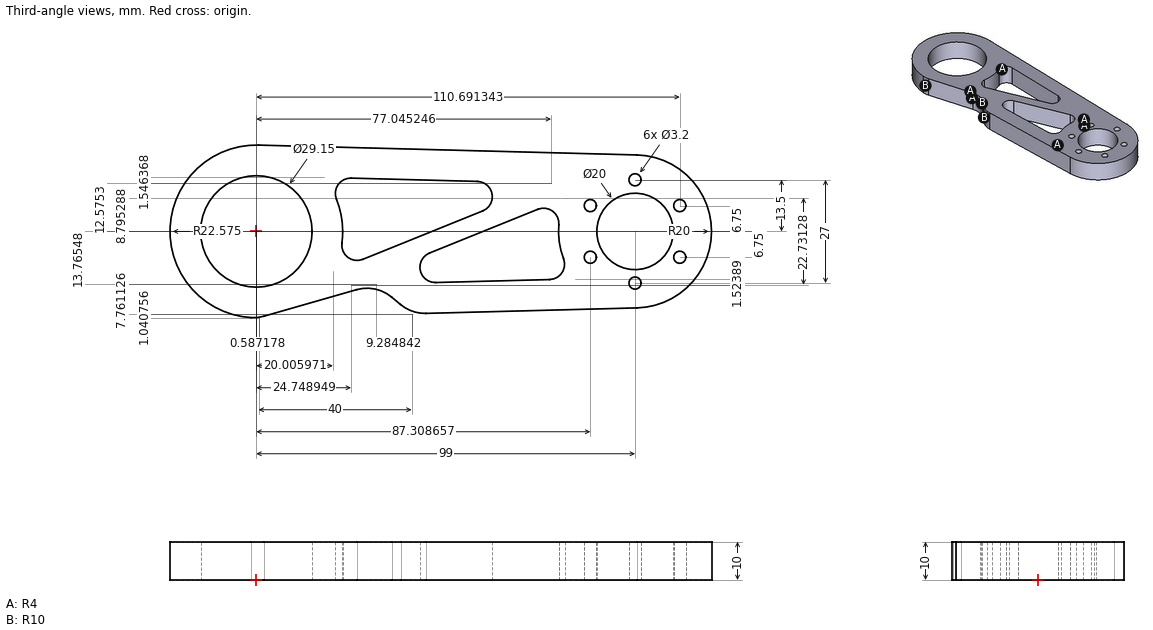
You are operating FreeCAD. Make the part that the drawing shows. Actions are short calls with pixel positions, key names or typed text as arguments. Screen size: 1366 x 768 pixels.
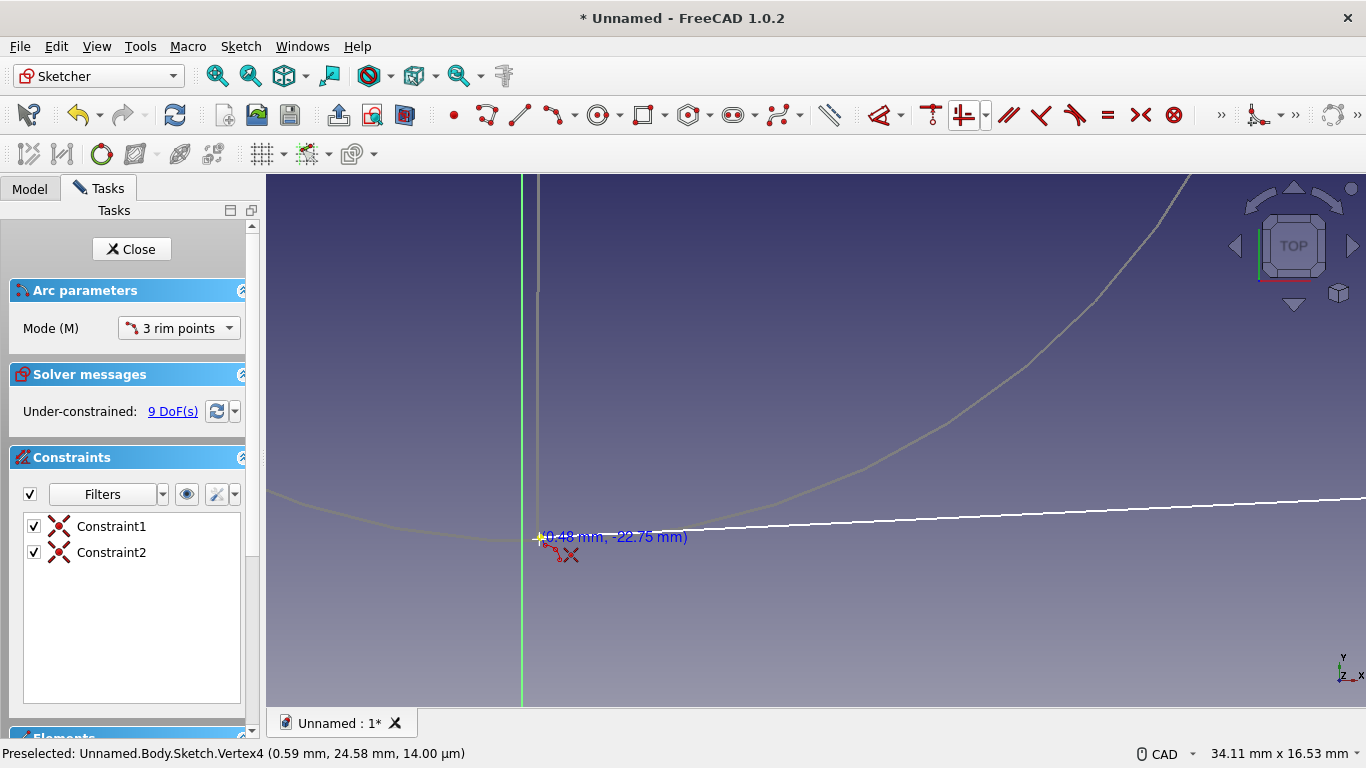
click(541, 537)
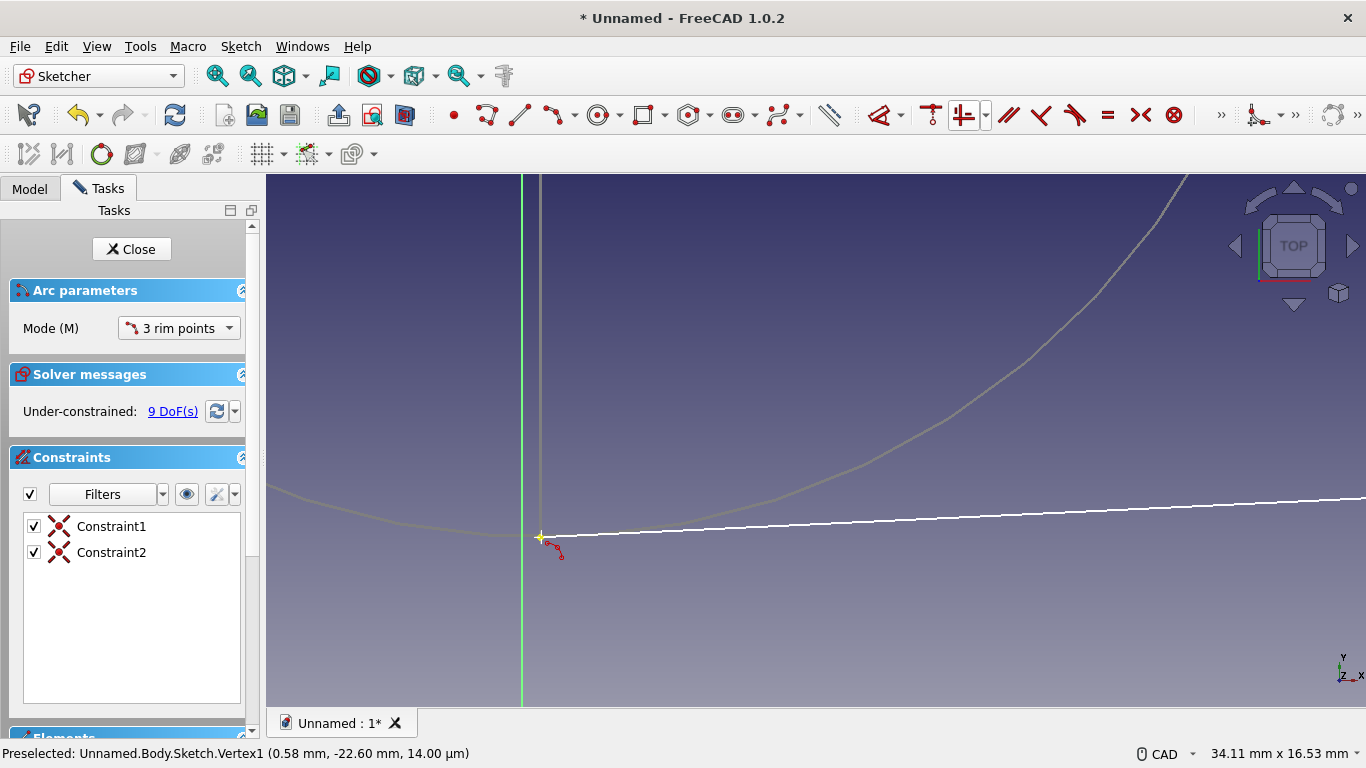
scroll(539, 539, down, 10)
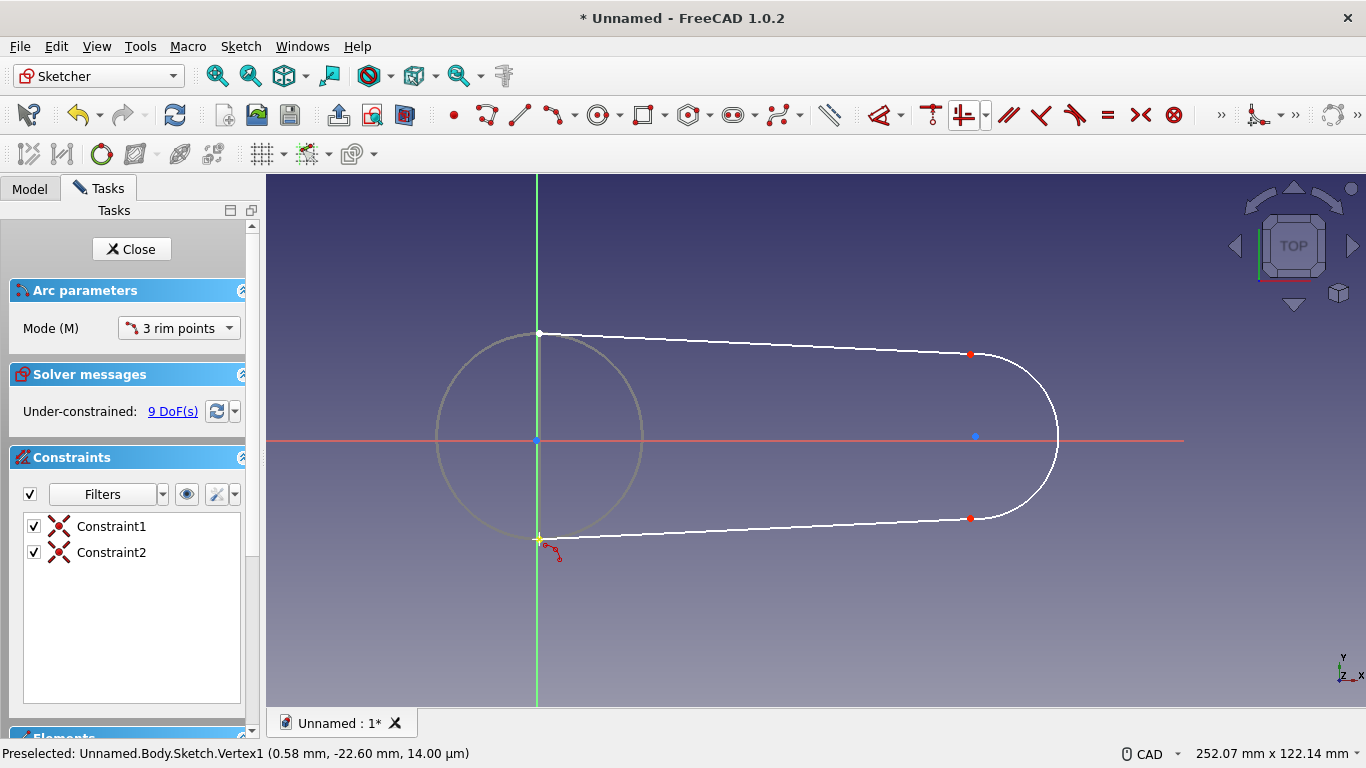
click(443, 410)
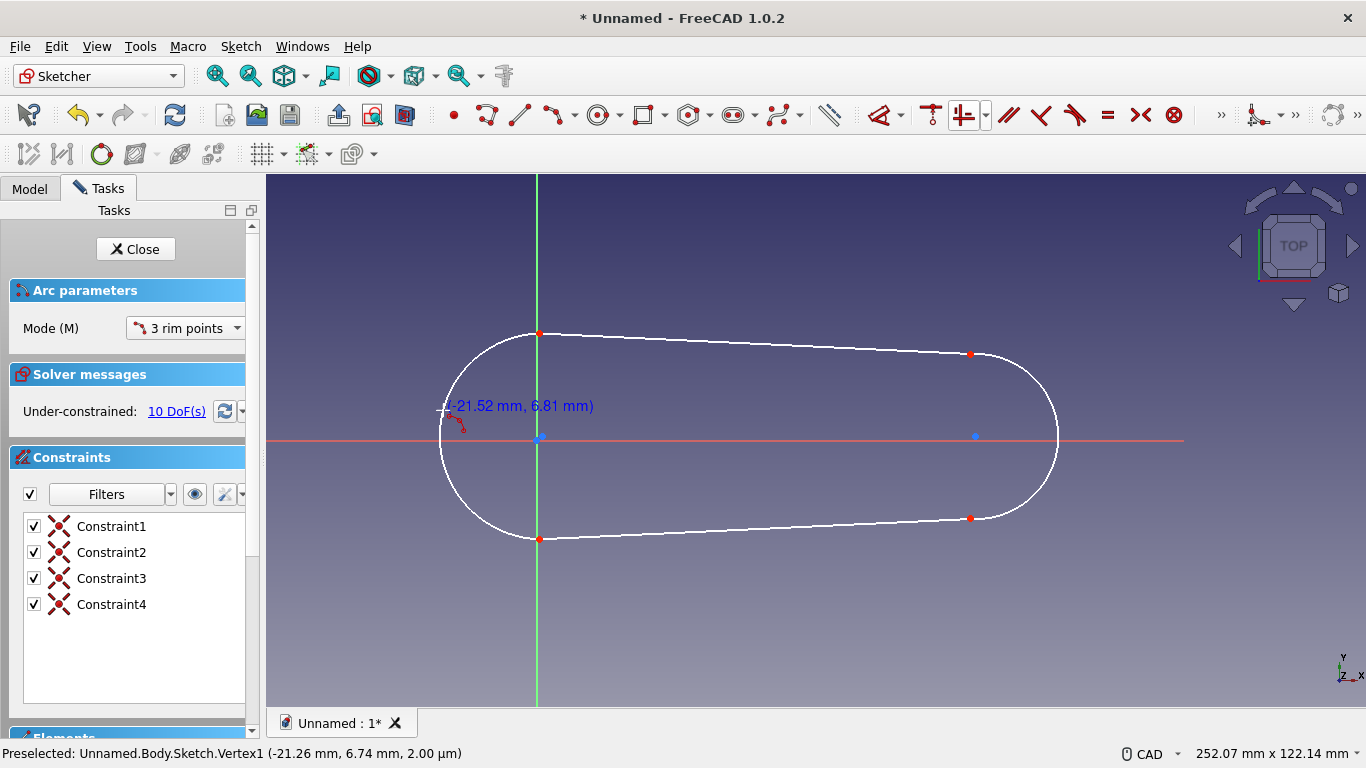
key(g)
key(c)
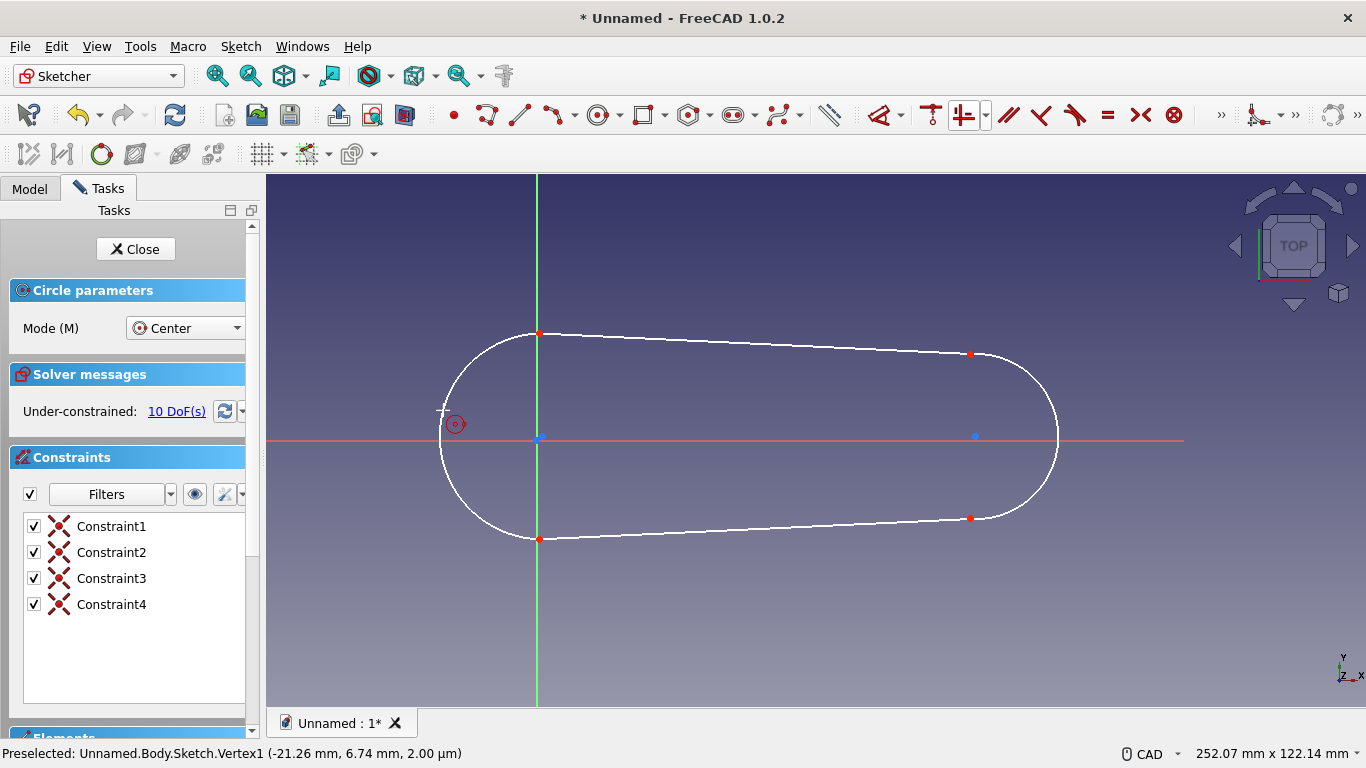
click(537, 441)
move(582, 396)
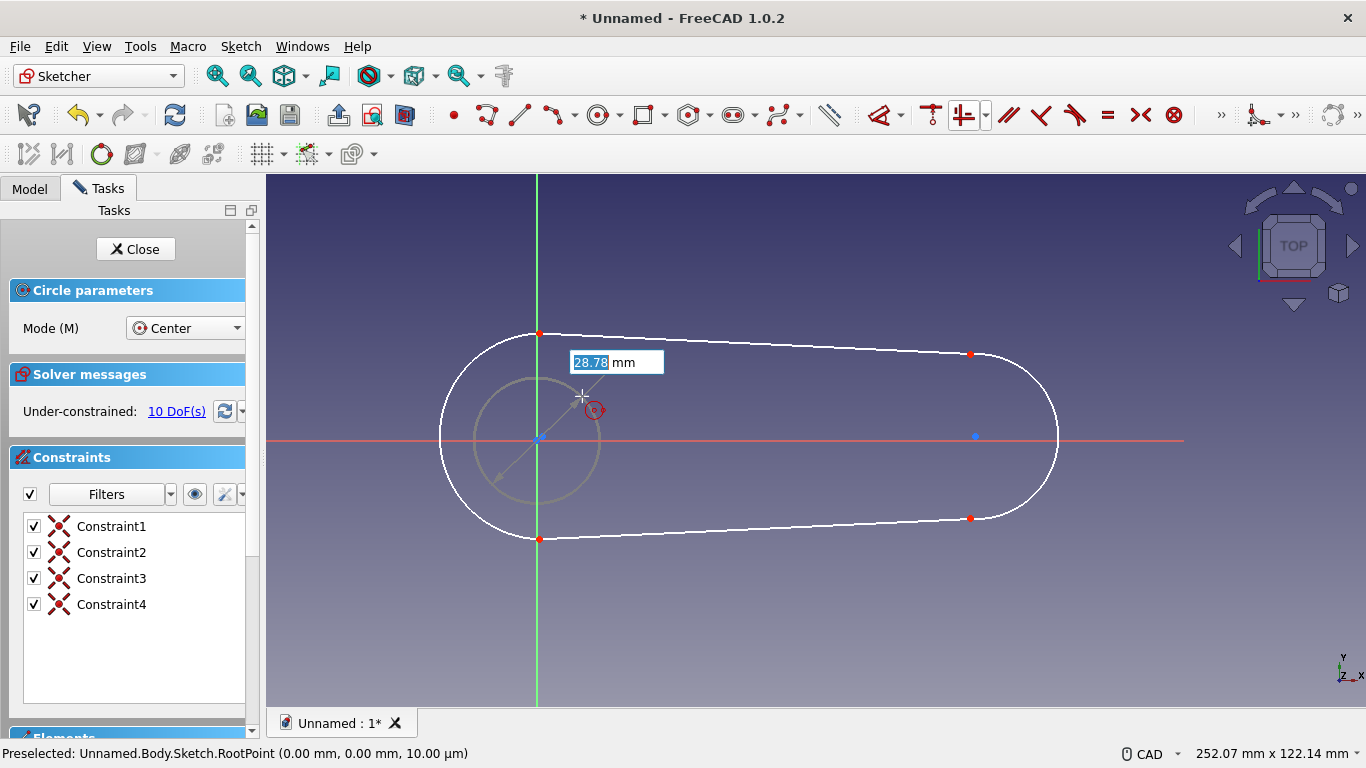
text(29.15)
key(Return)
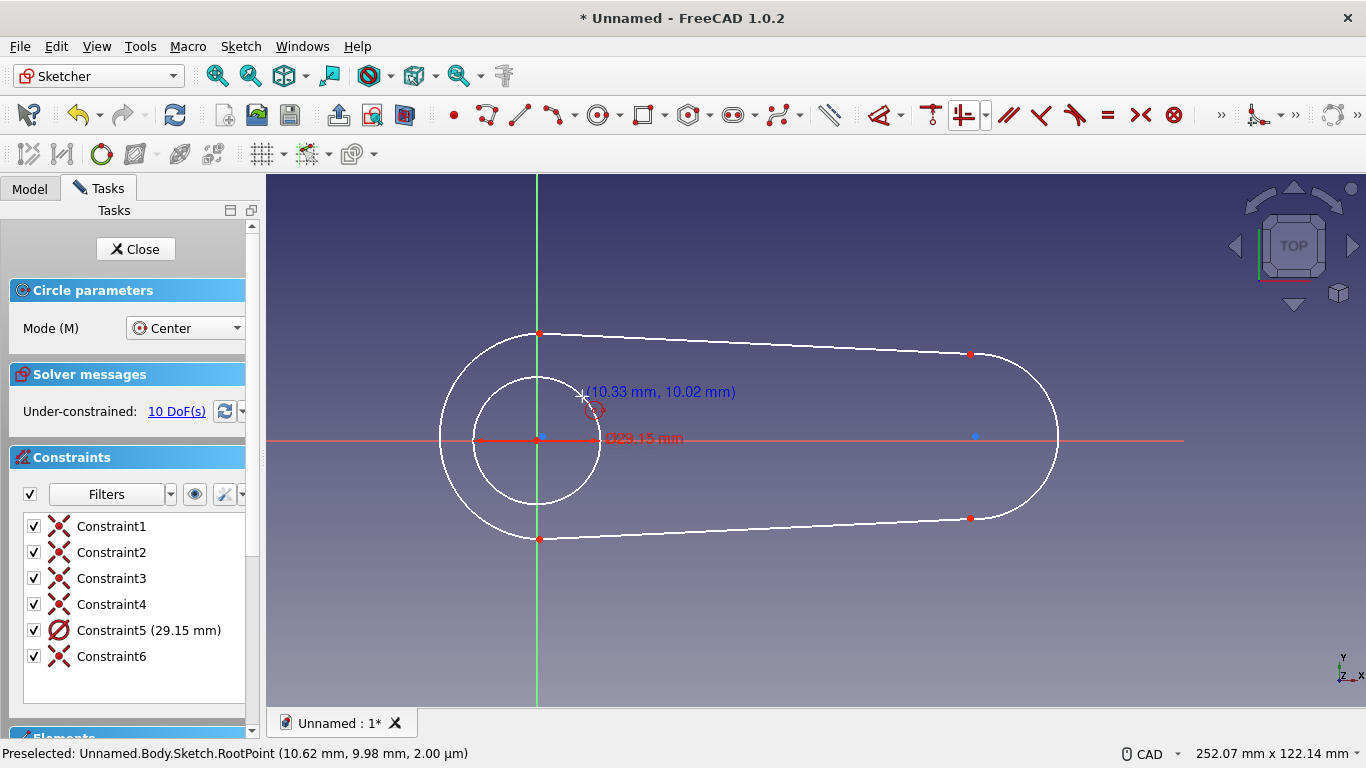
click(969, 441)
move(1000, 410)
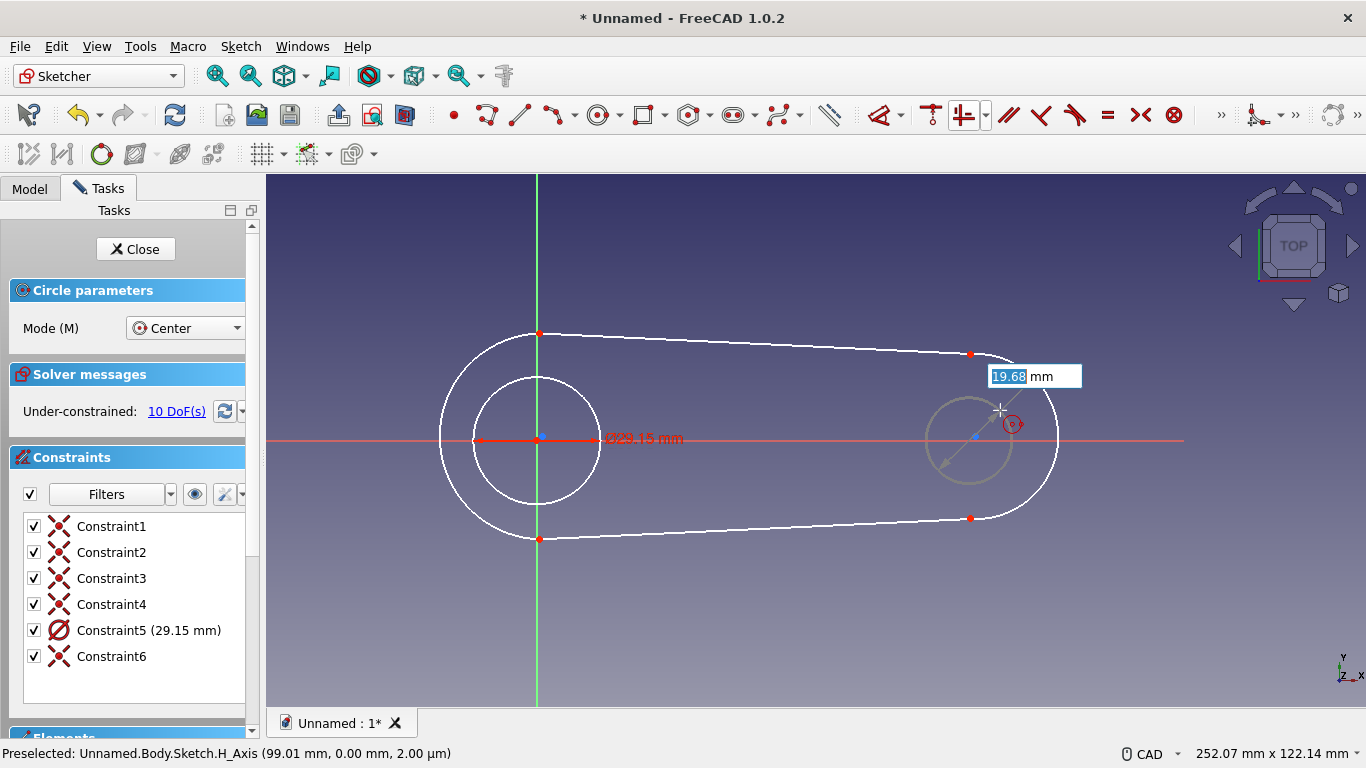
text(20)
key(Return)
key(Escape)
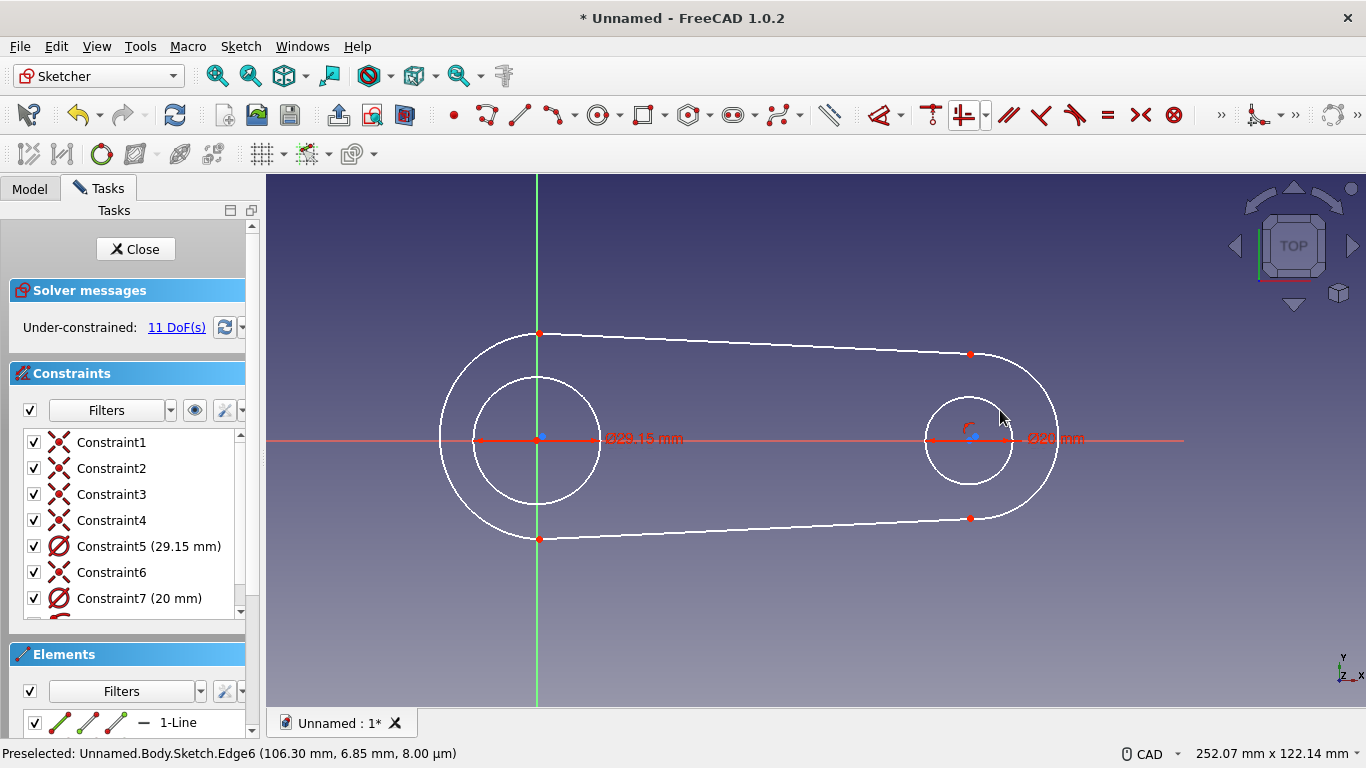
click(669, 533)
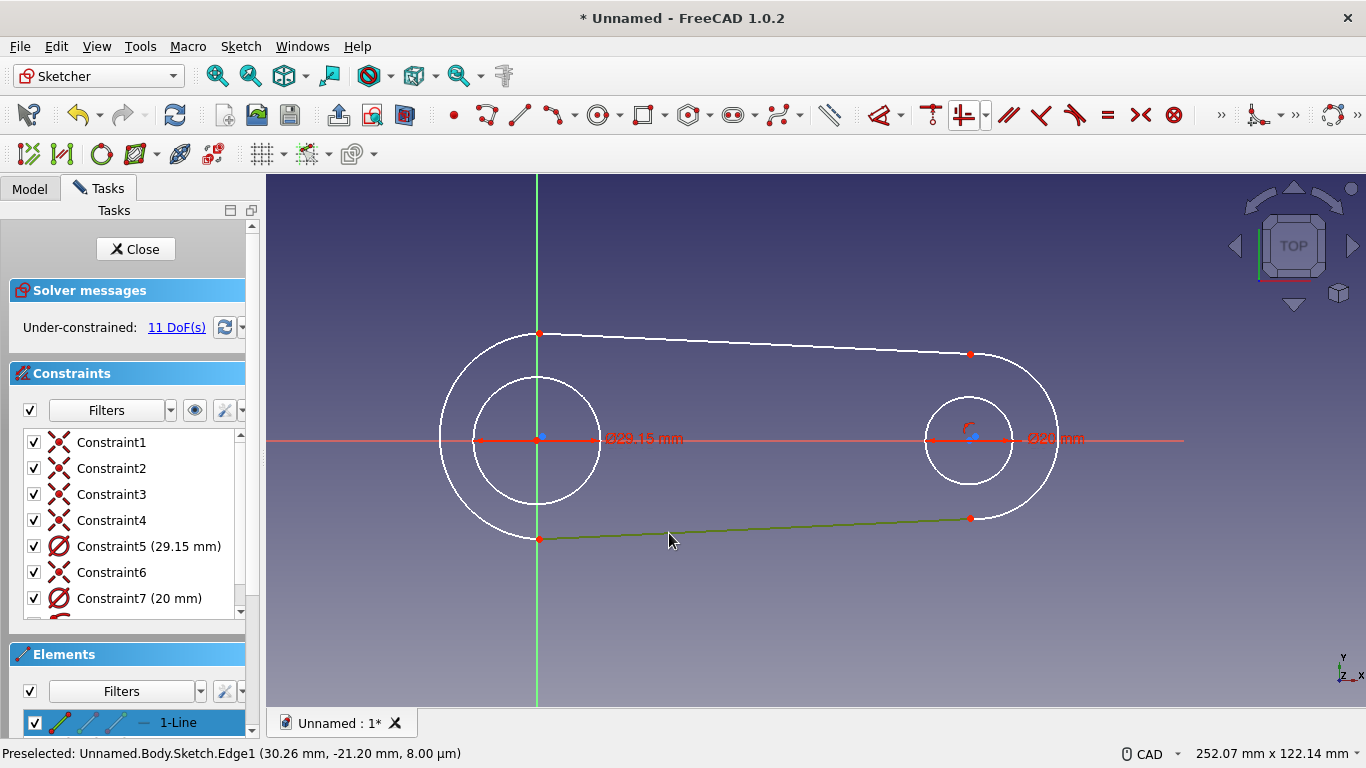
click(1041, 487)